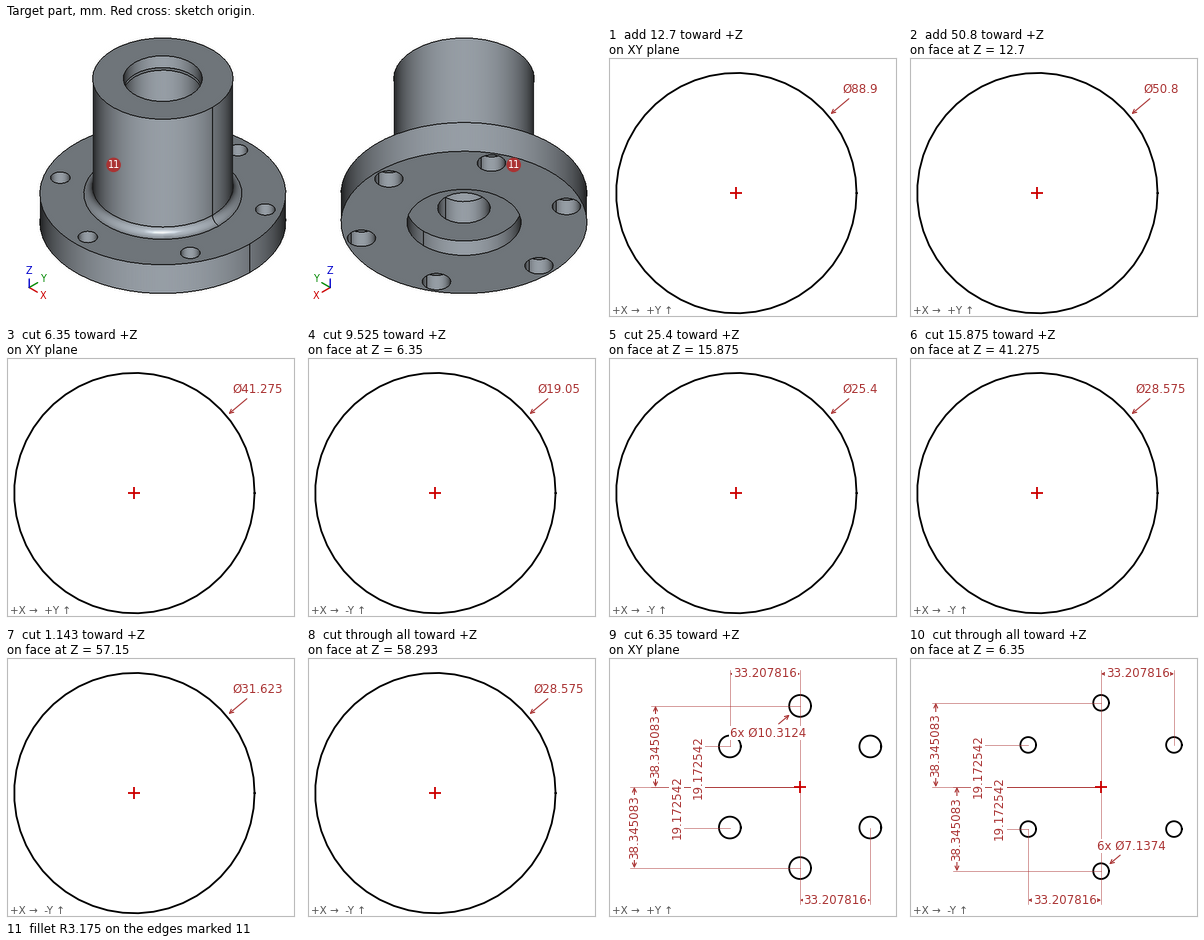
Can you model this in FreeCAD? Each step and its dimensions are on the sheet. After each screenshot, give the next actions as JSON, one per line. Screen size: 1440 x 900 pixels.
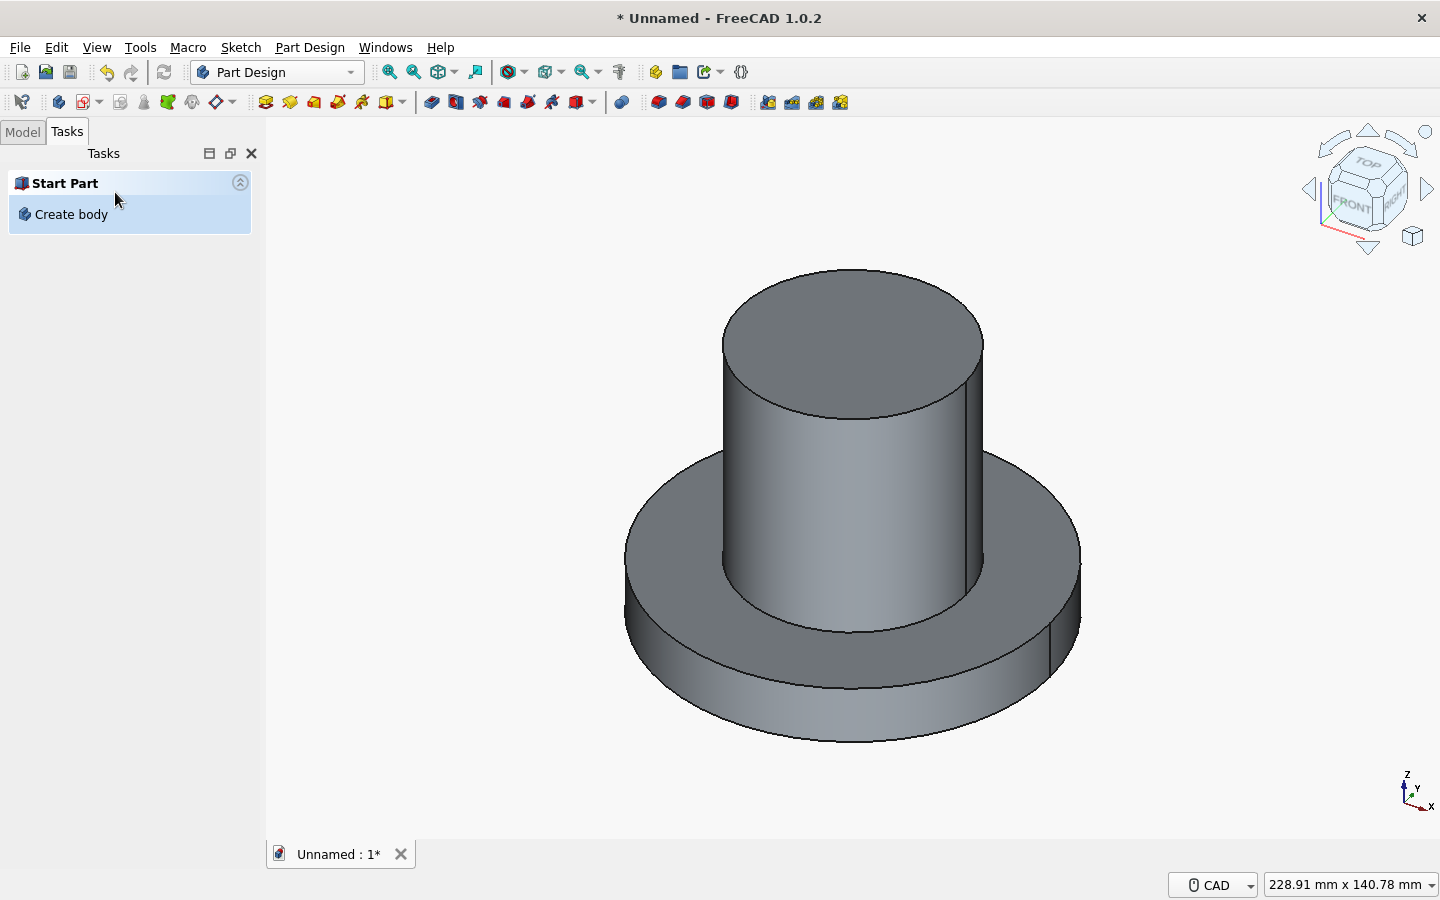
{"action": "key", "text": "5"}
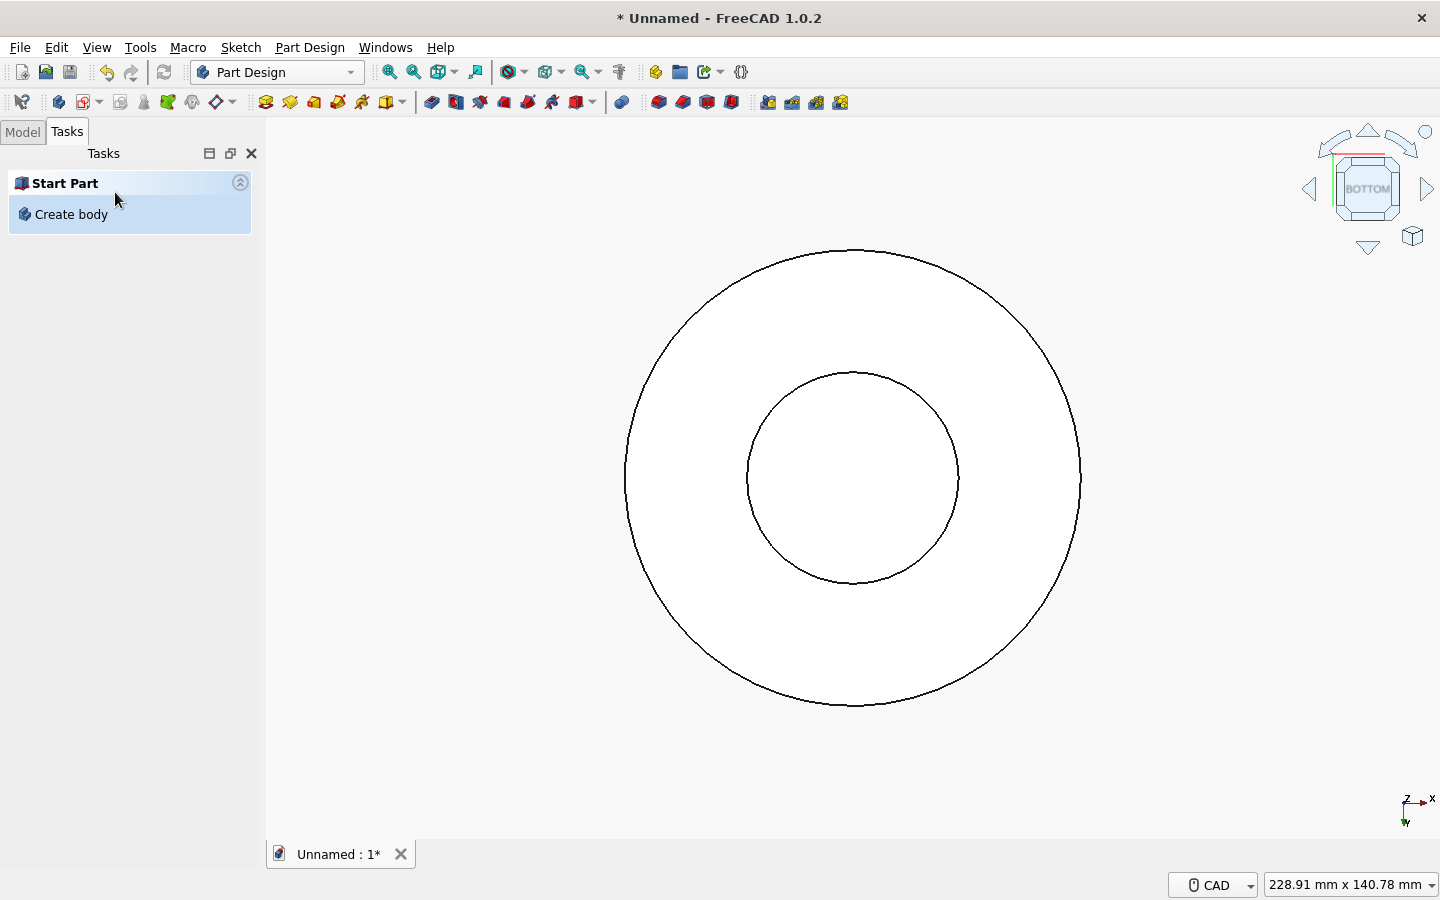
{"action": "left_click", "coordinate": [853, 477]}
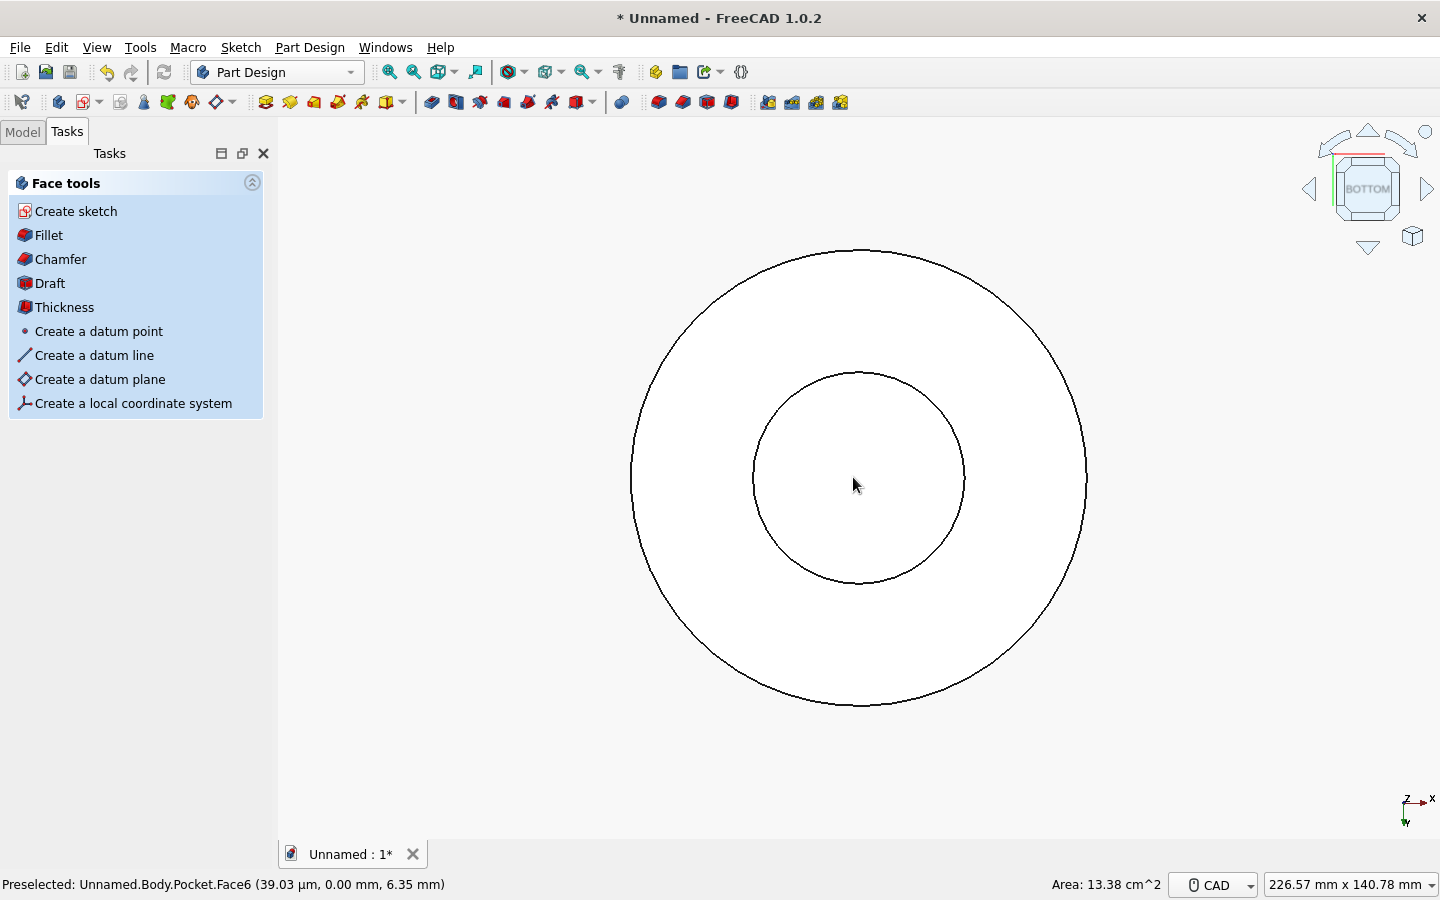
{"action": "left_click", "coordinate": [84, 102]}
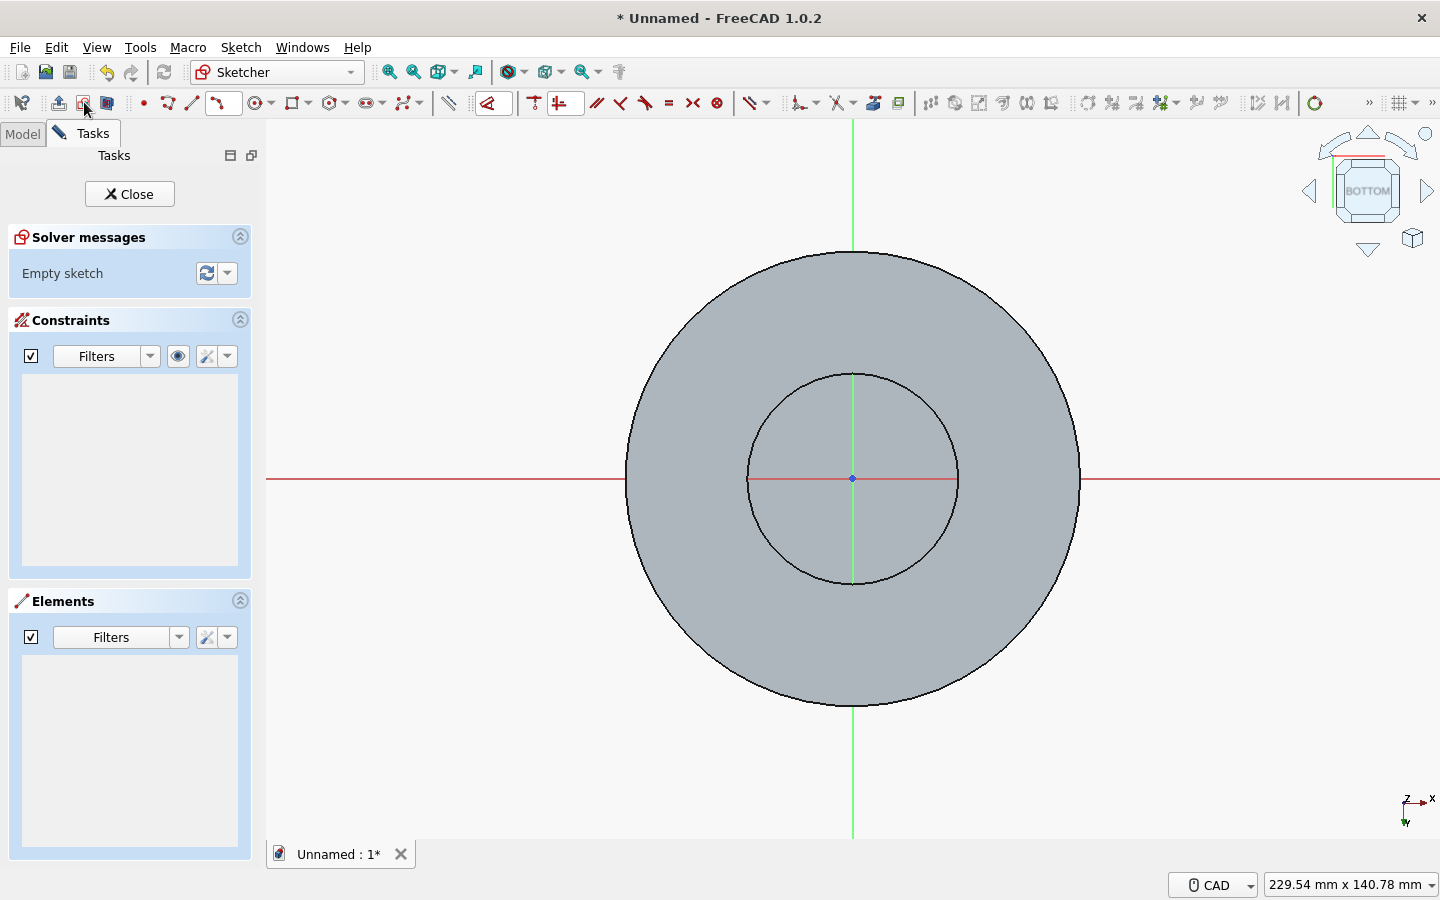
{"action": "scroll", "coordinate": [870, 479], "scroll_direction": "up", "scroll_amount": 8}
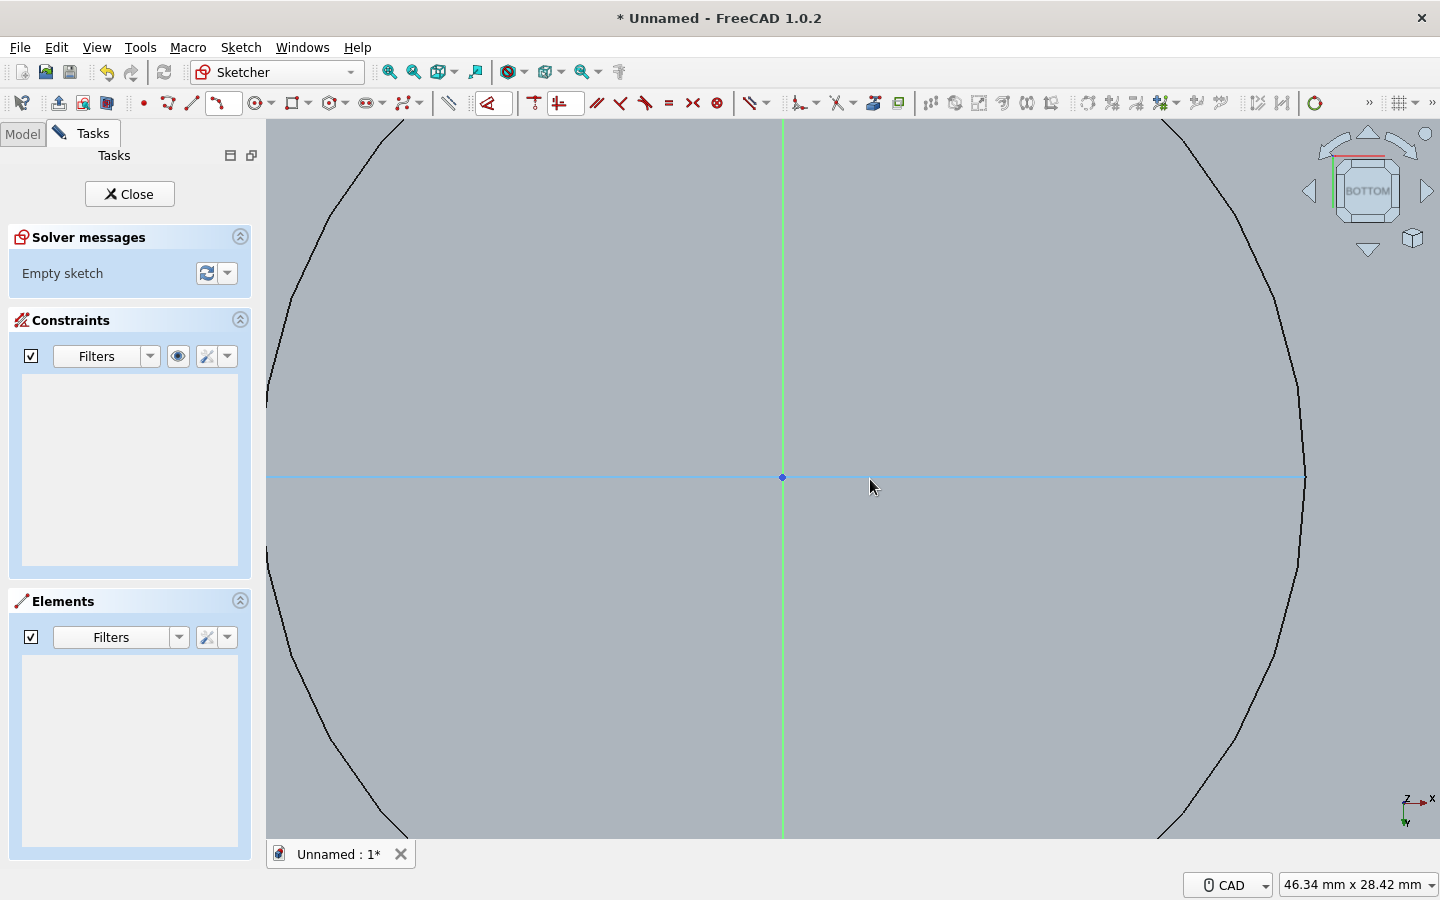
{"action": "left_click", "coordinate": [256, 104]}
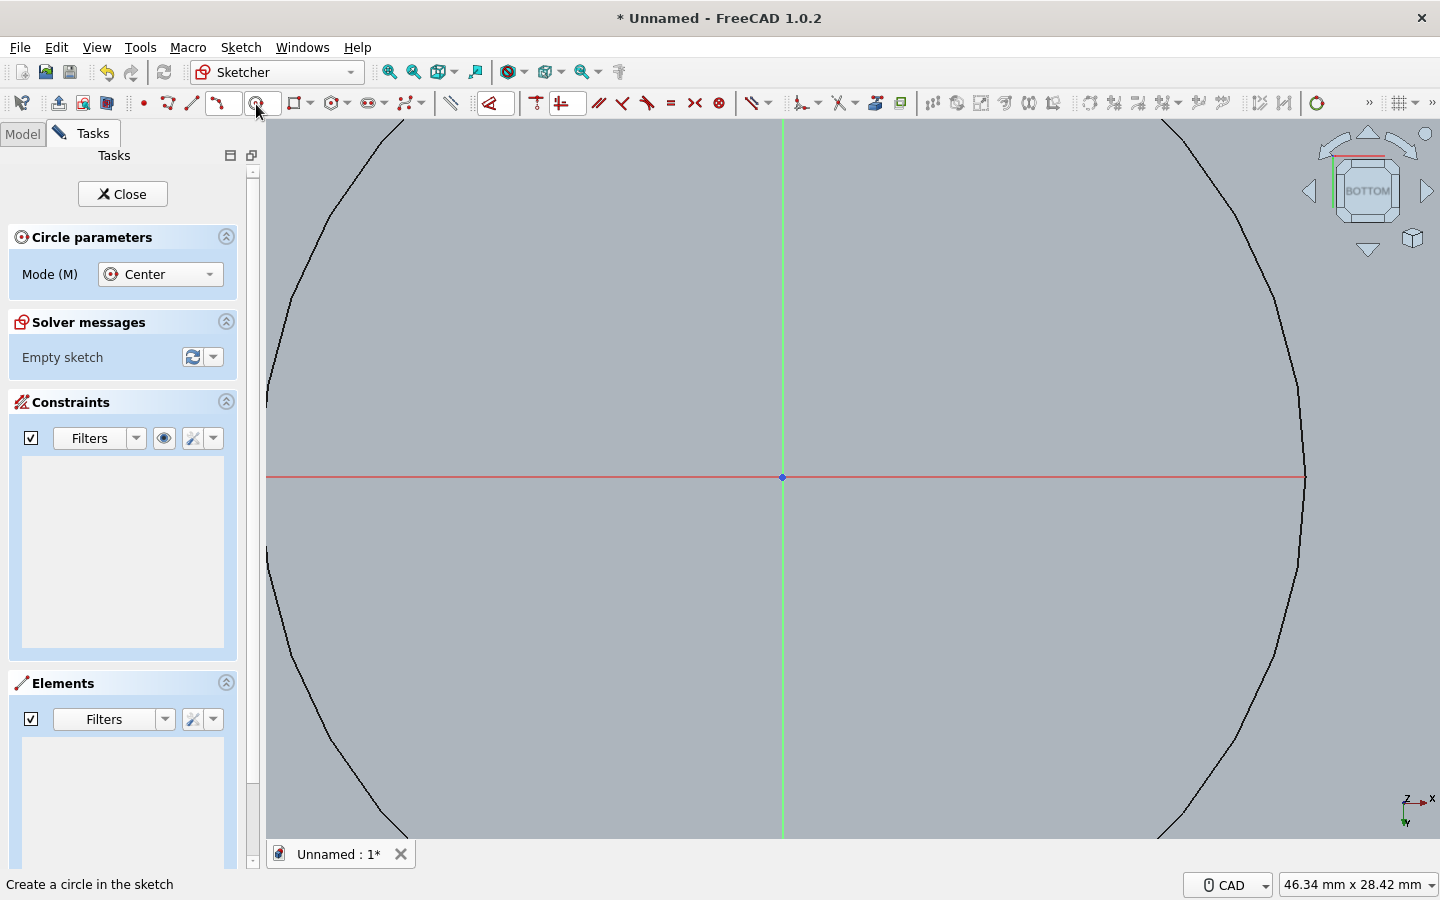
{"action": "left_click", "coordinate": [783, 477]}
{"action": "mouse_move", "coordinate": [953, 306]}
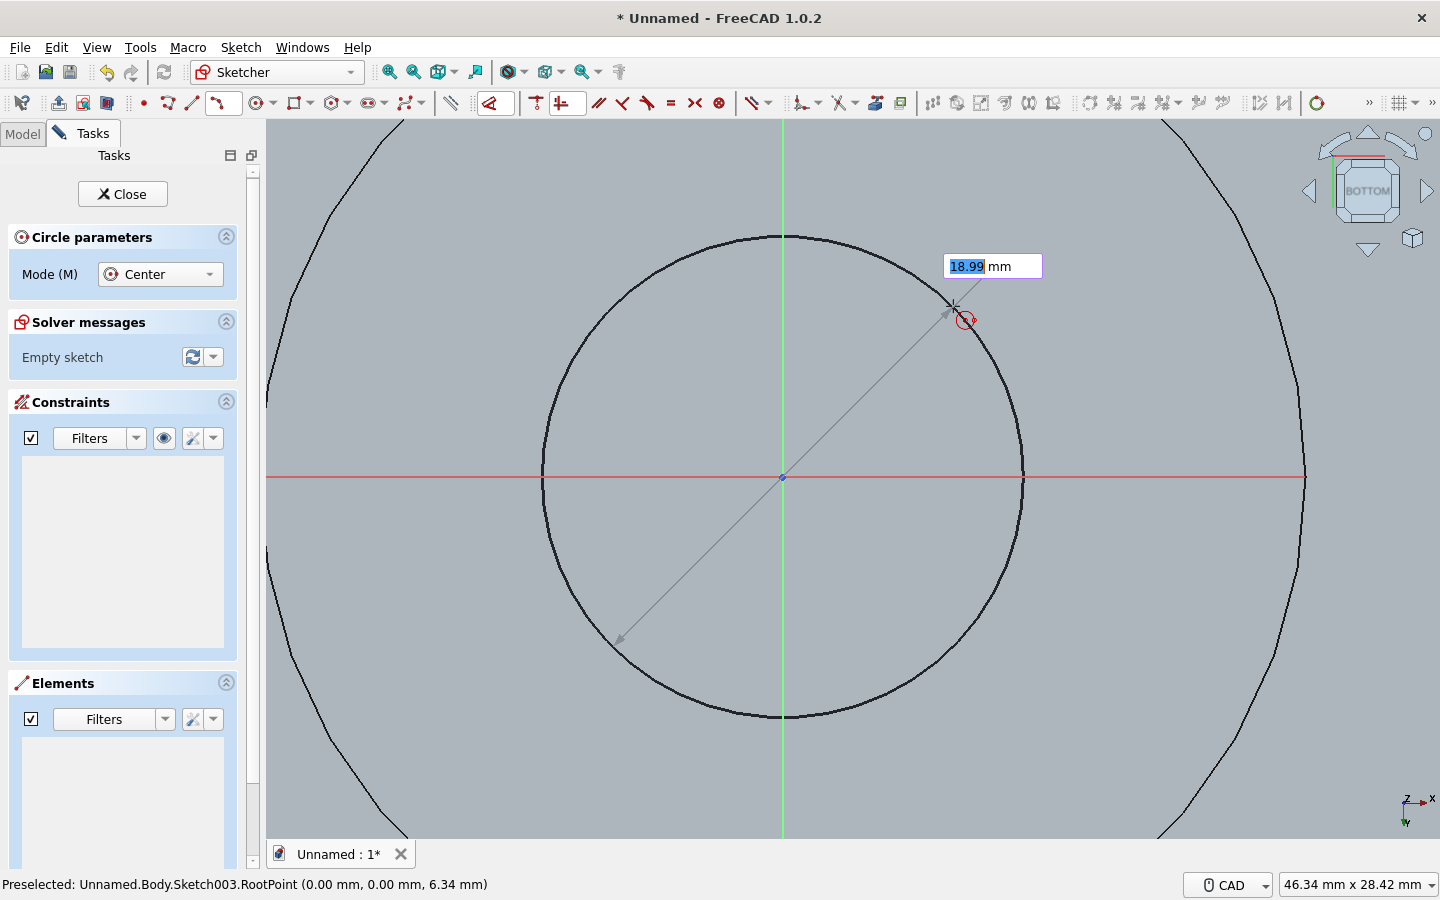
{"action": "type", "text": "19.05"}
{"action": "key", "text": "Return"}
{"action": "key", "text": "Escape"}